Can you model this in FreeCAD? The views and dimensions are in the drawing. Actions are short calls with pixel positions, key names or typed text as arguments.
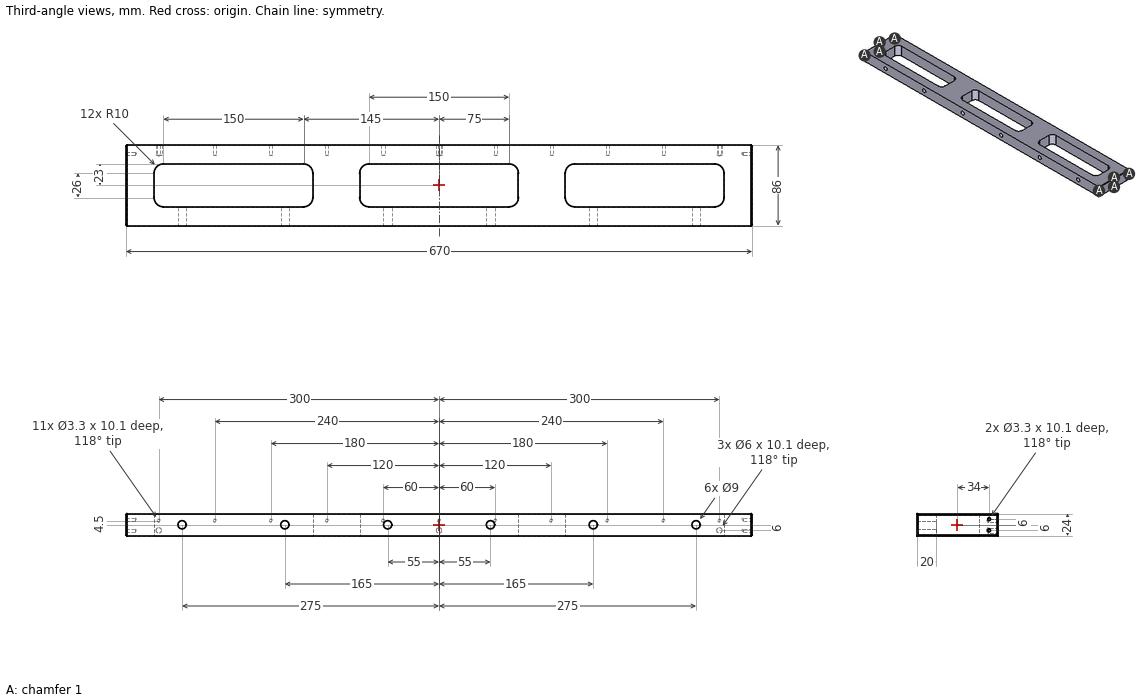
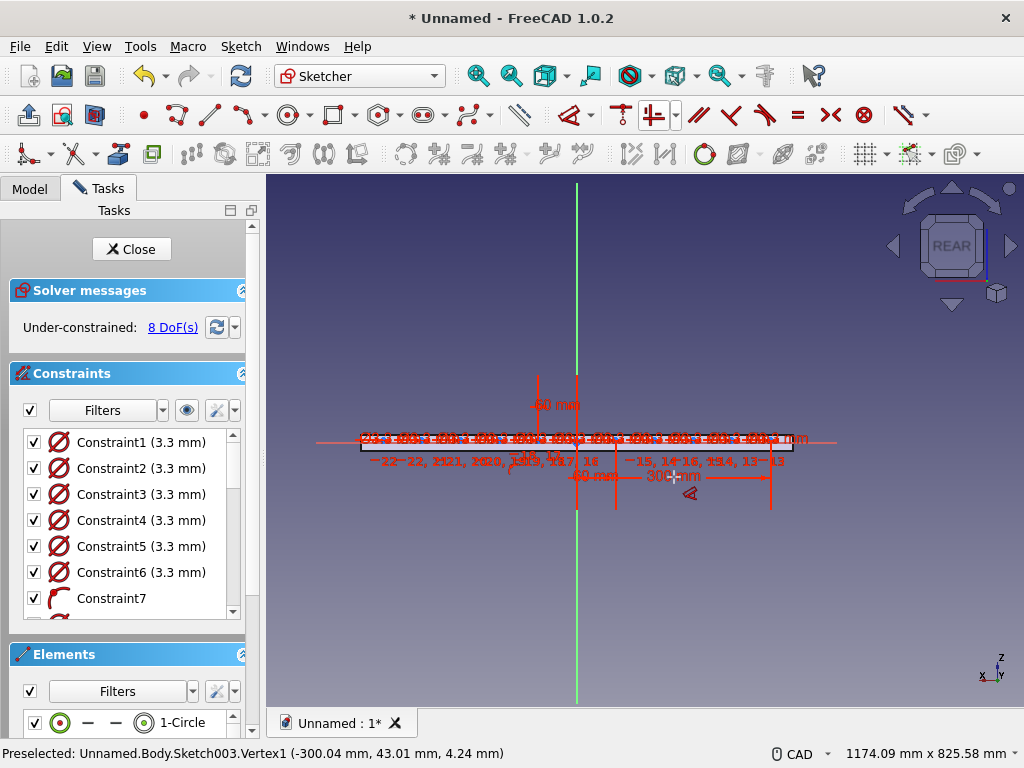
scroll(771, 440, up, 14)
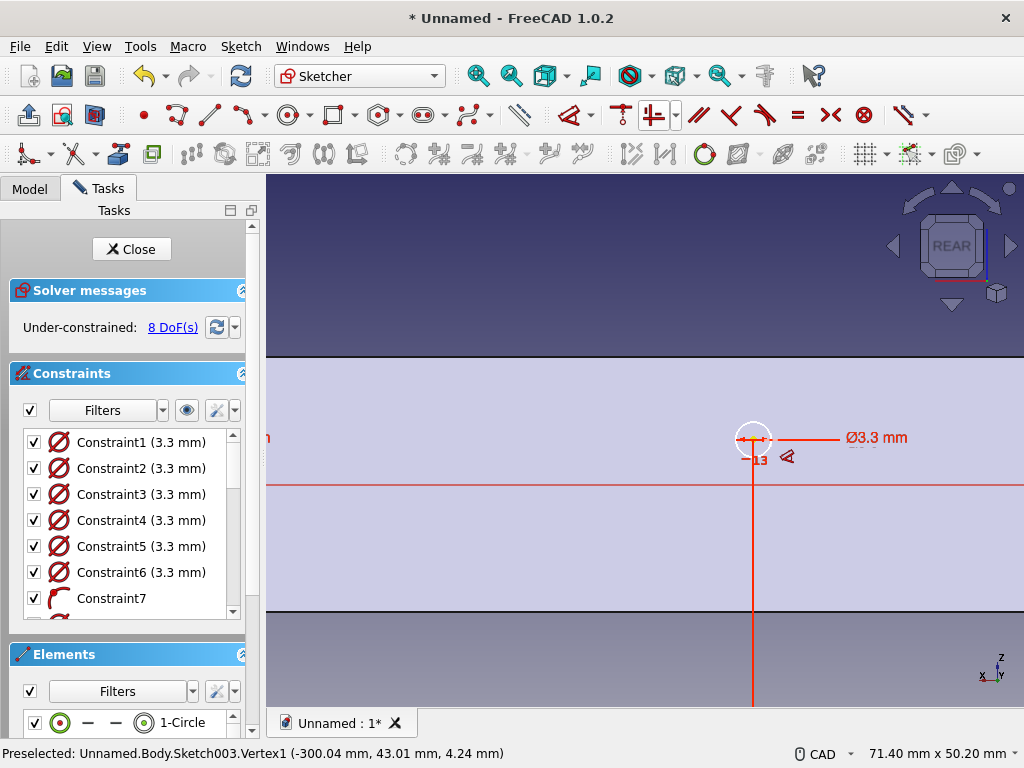
click(753, 440)
click(787, 462)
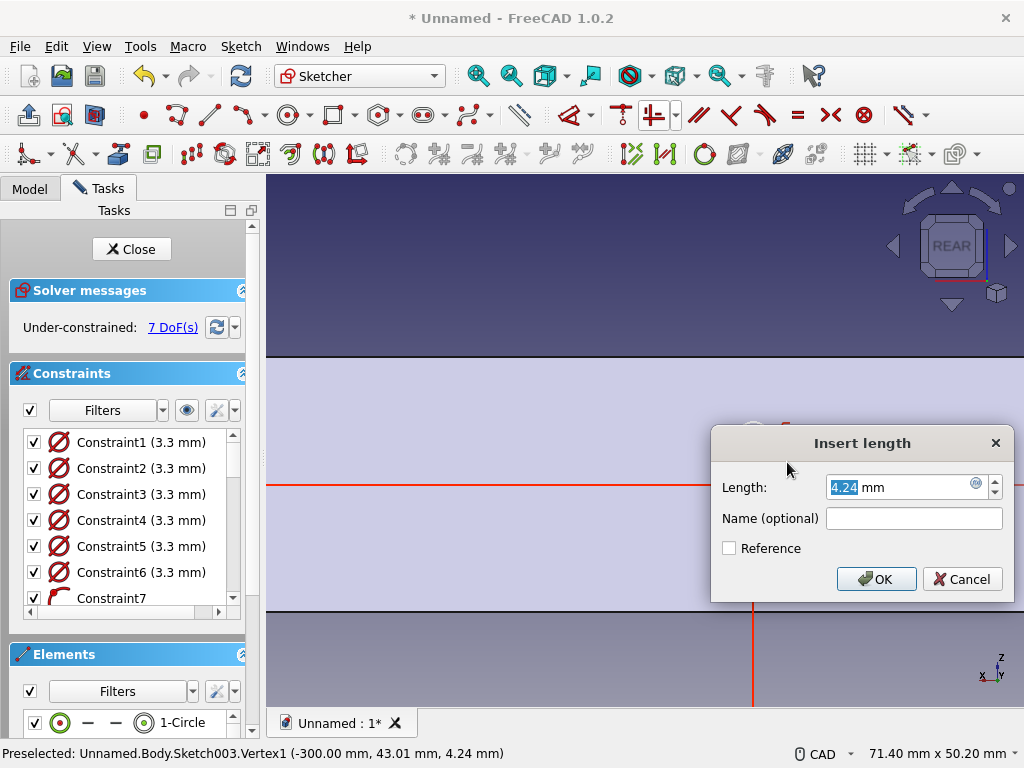
text(4.5)
key(Return)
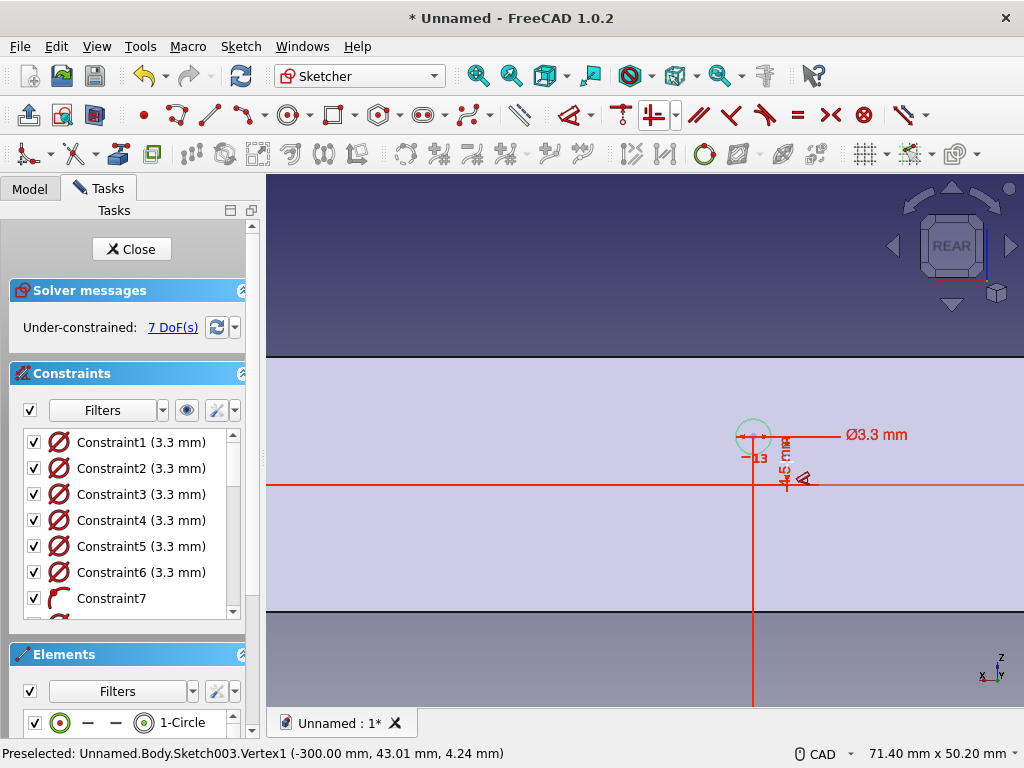
scroll(771, 440, down, 14)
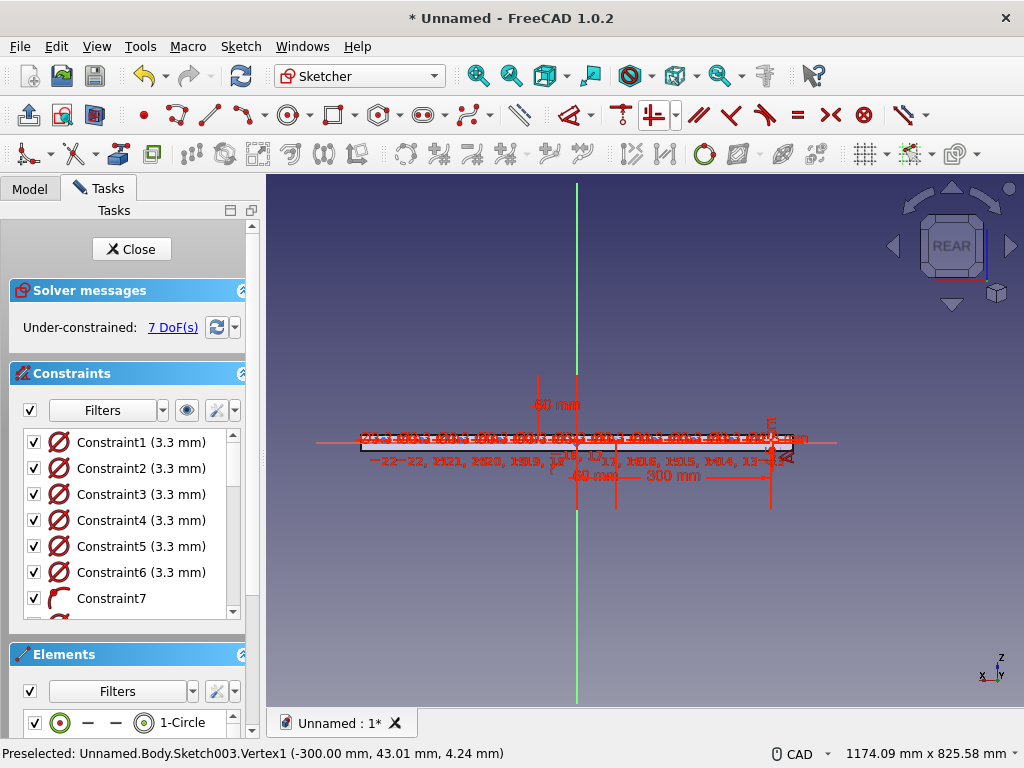
click(732, 440)
click(654, 406)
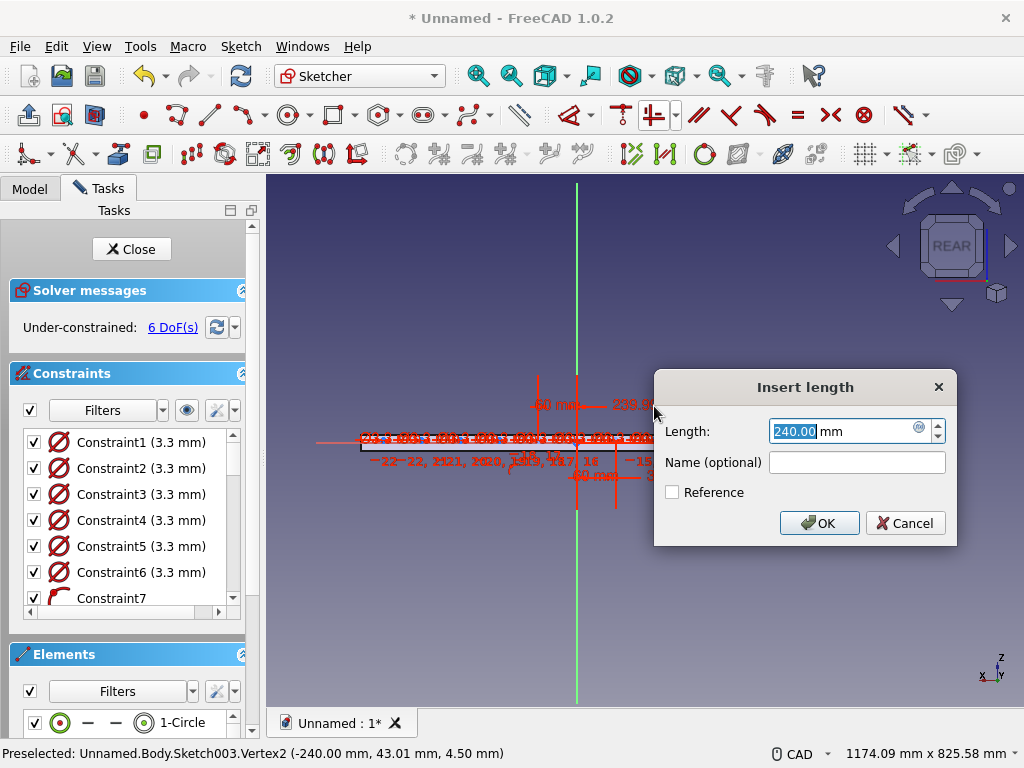
text(240)
key(Return)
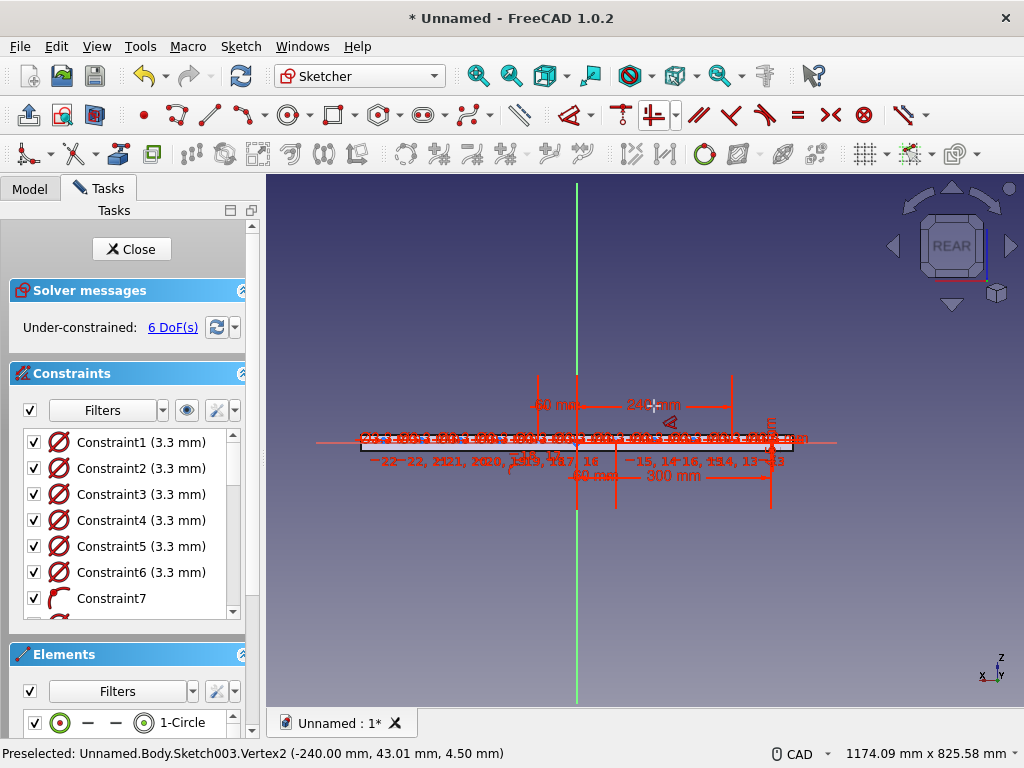
click(693, 440)
click(635, 501)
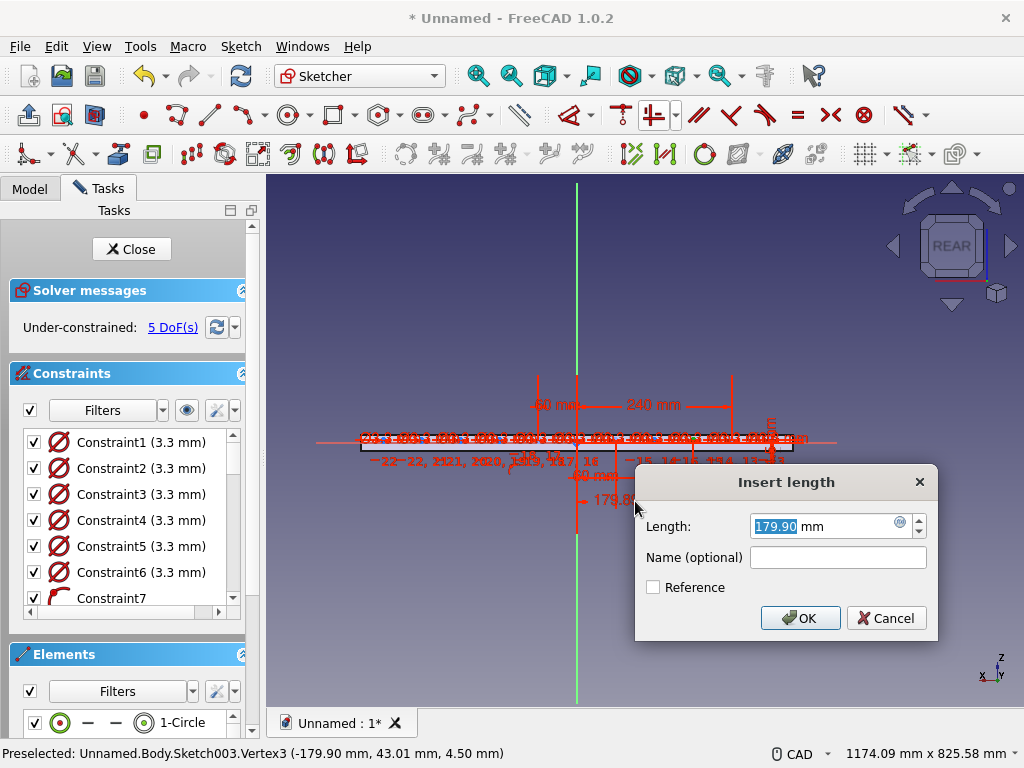
text(180)
key(Return)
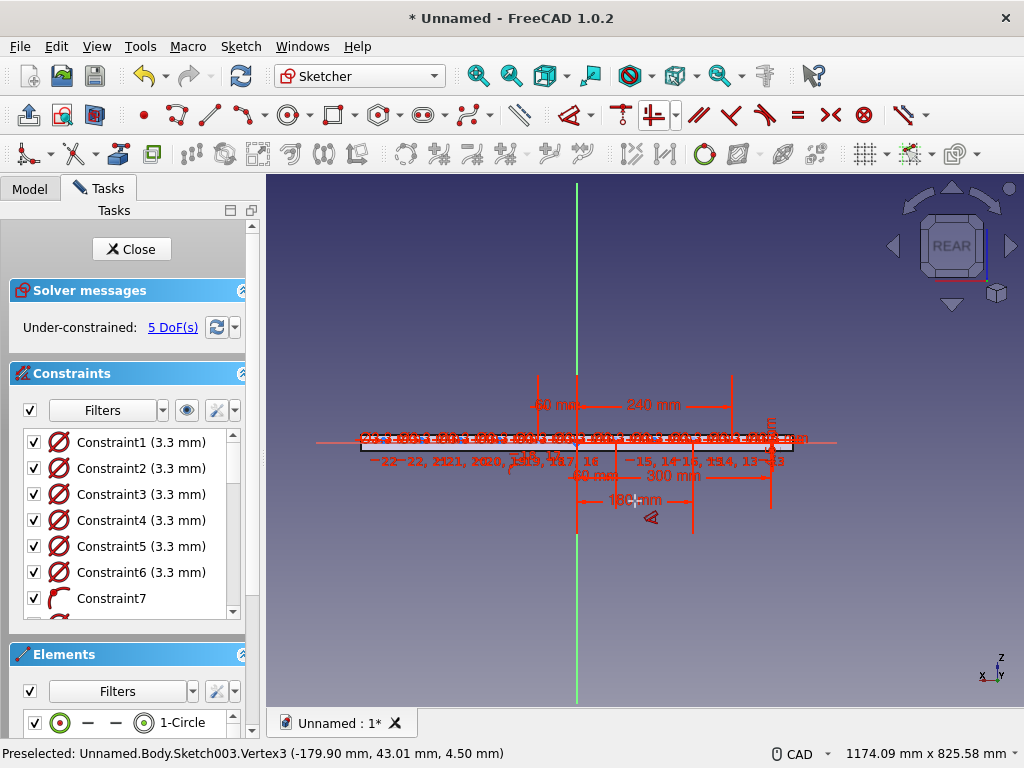
click(654, 440)
click(616, 382)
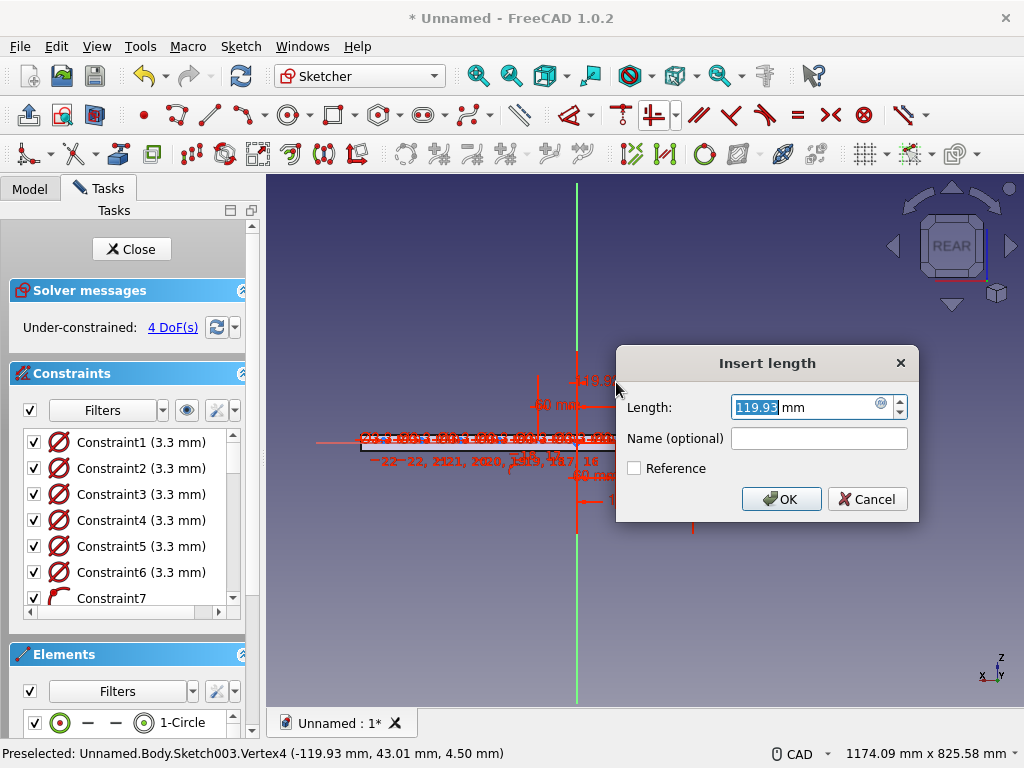
text(120)
key(Return)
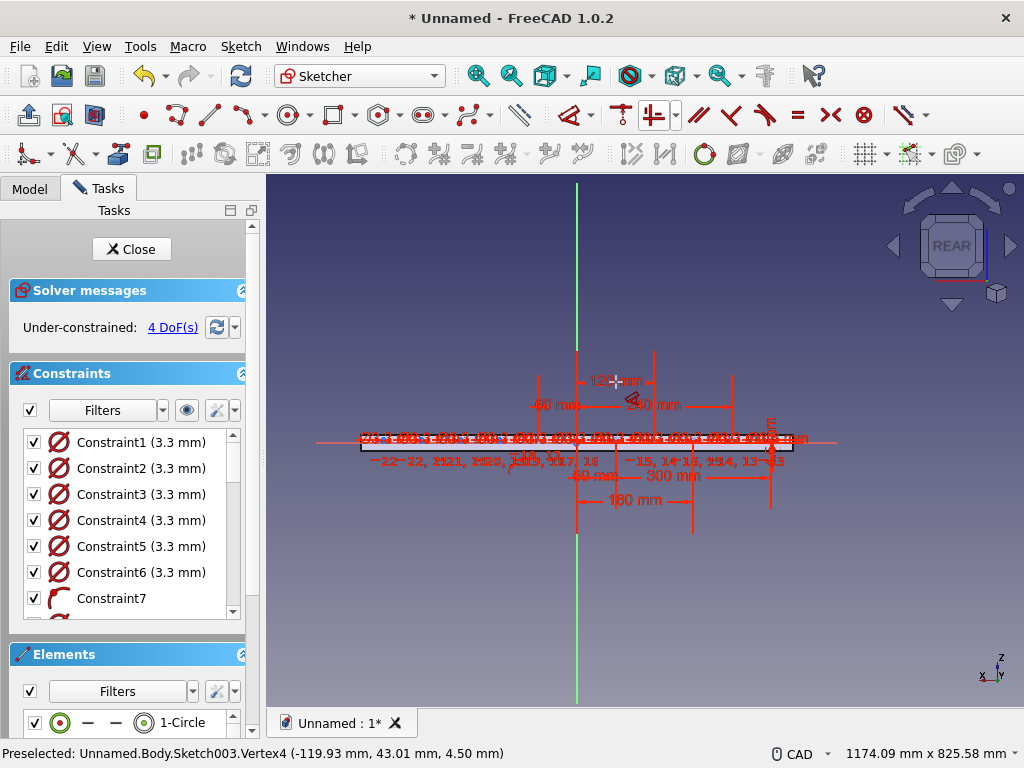
click(499, 440)
click(520, 477)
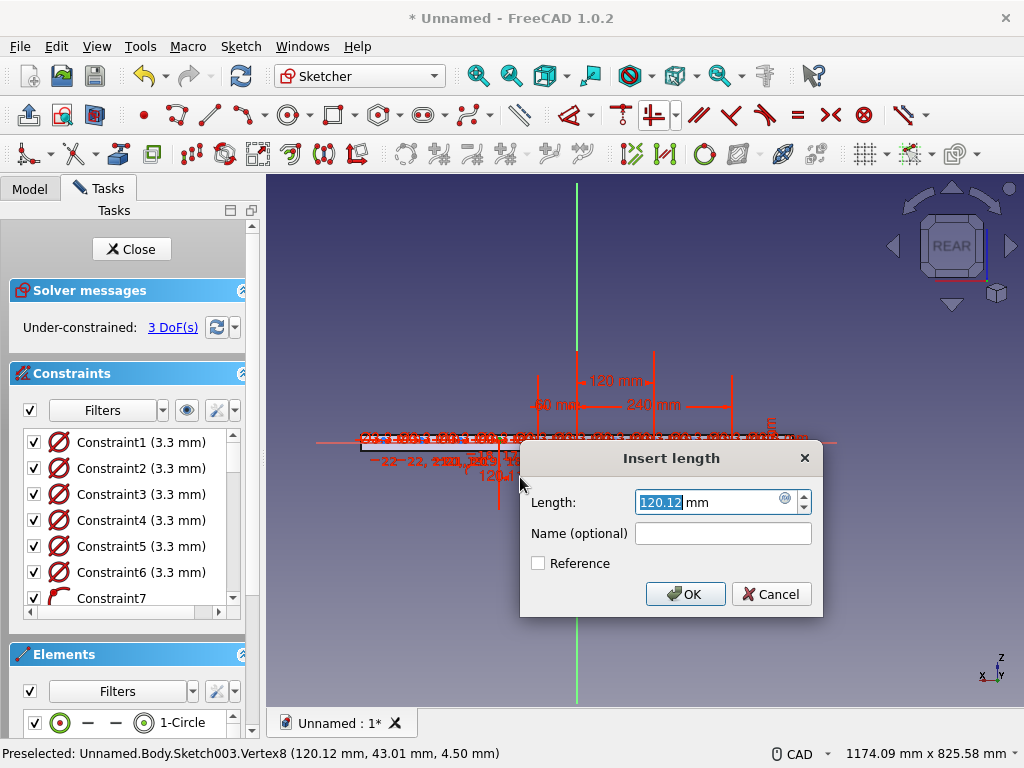
text(120)
key(Return)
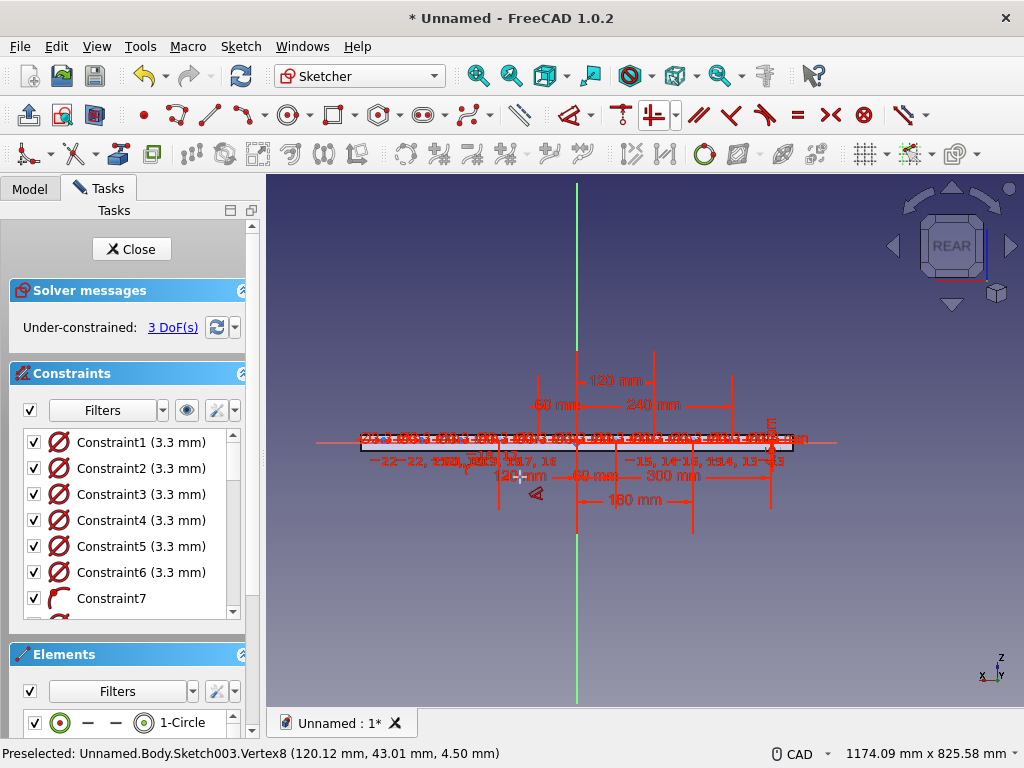
click(461, 440)
click(478, 406)